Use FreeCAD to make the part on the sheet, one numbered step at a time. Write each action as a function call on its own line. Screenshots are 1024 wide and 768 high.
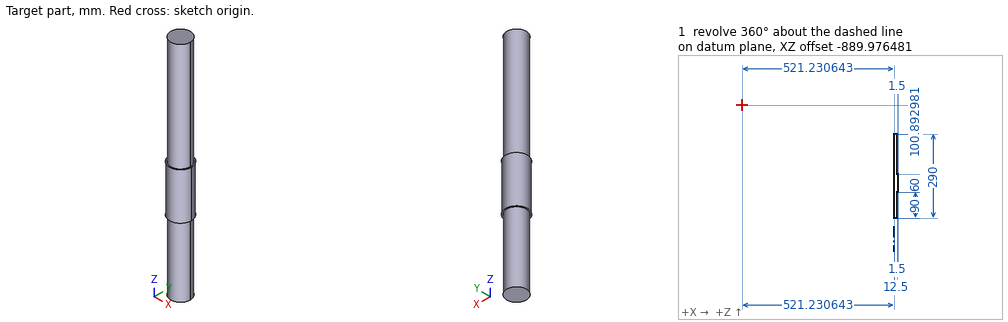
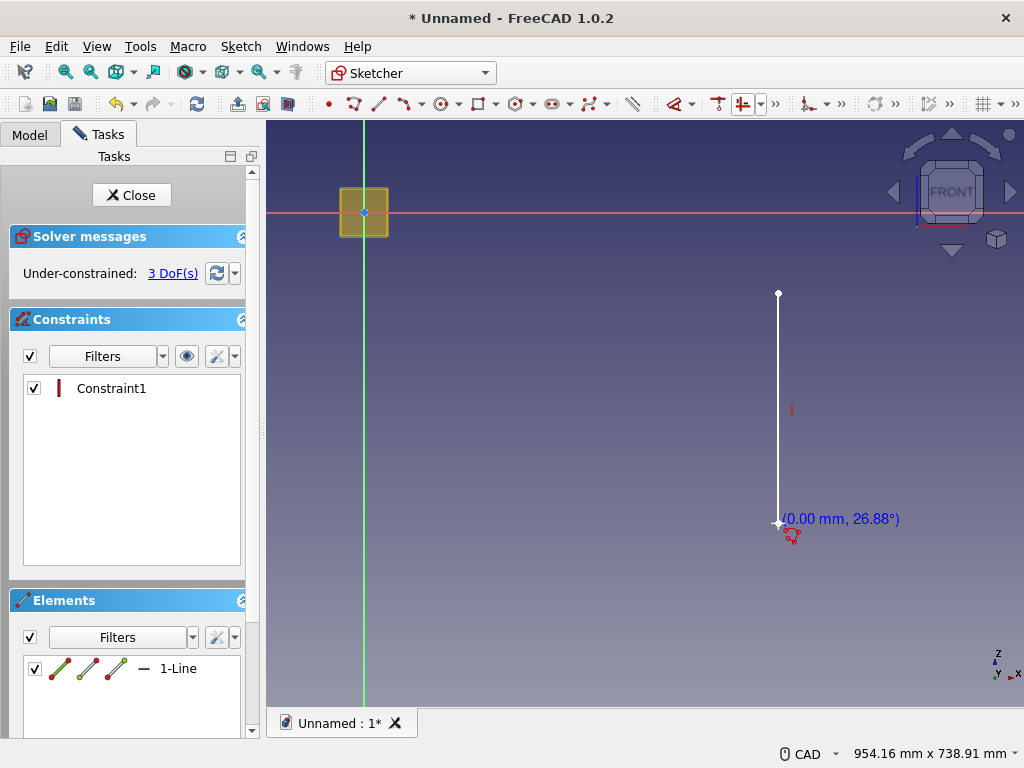
scroll(788, 523, up, 3)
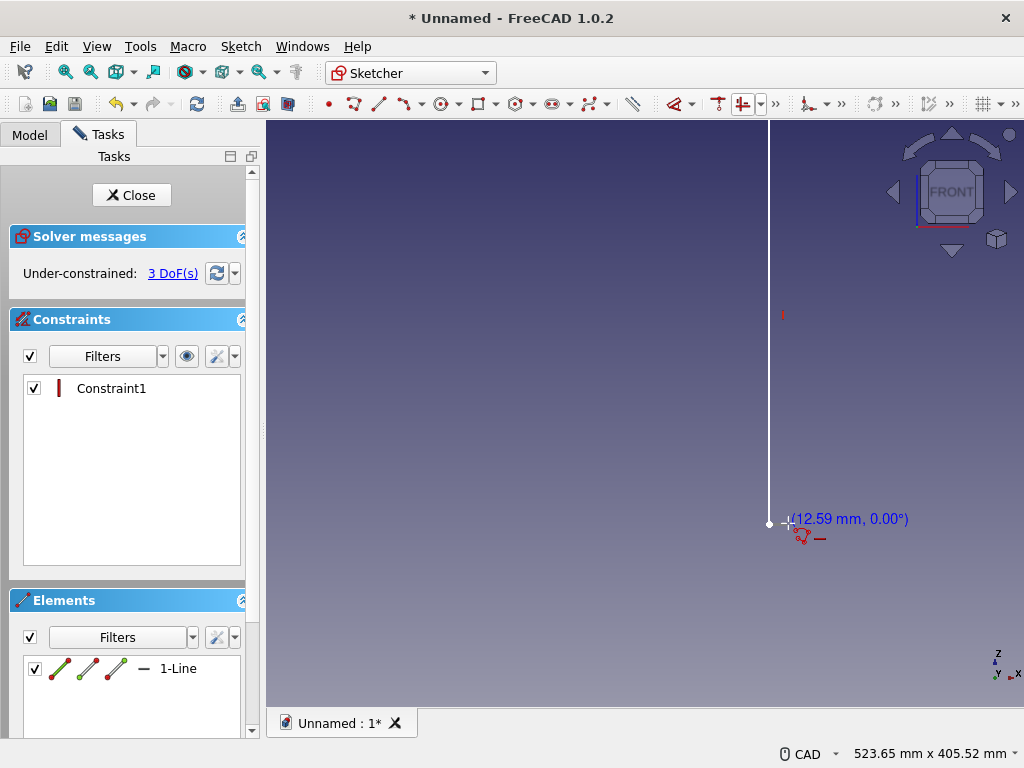
click(788, 522)
click(788, 392)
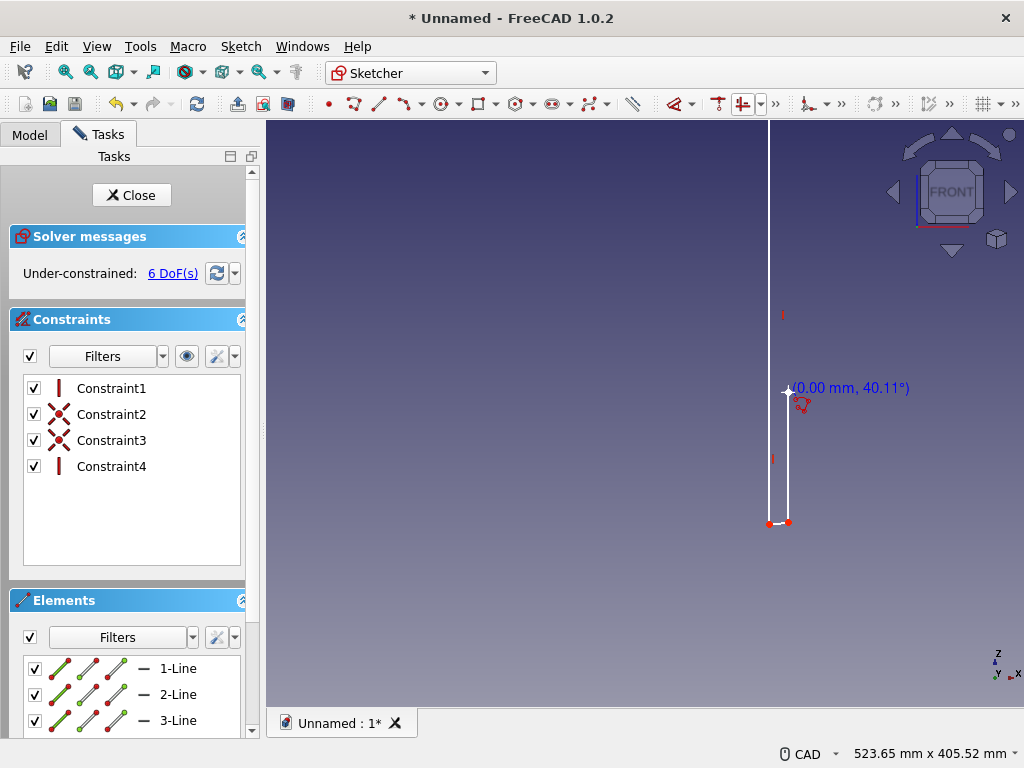
scroll(790, 392, up, 10)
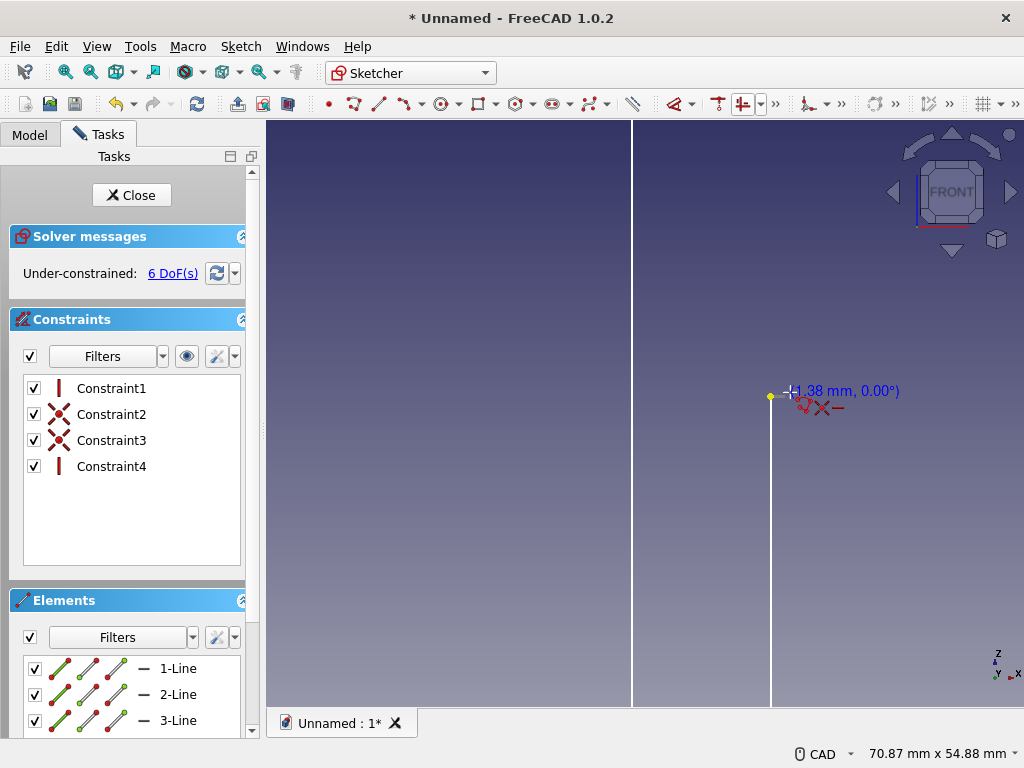
click(783, 389)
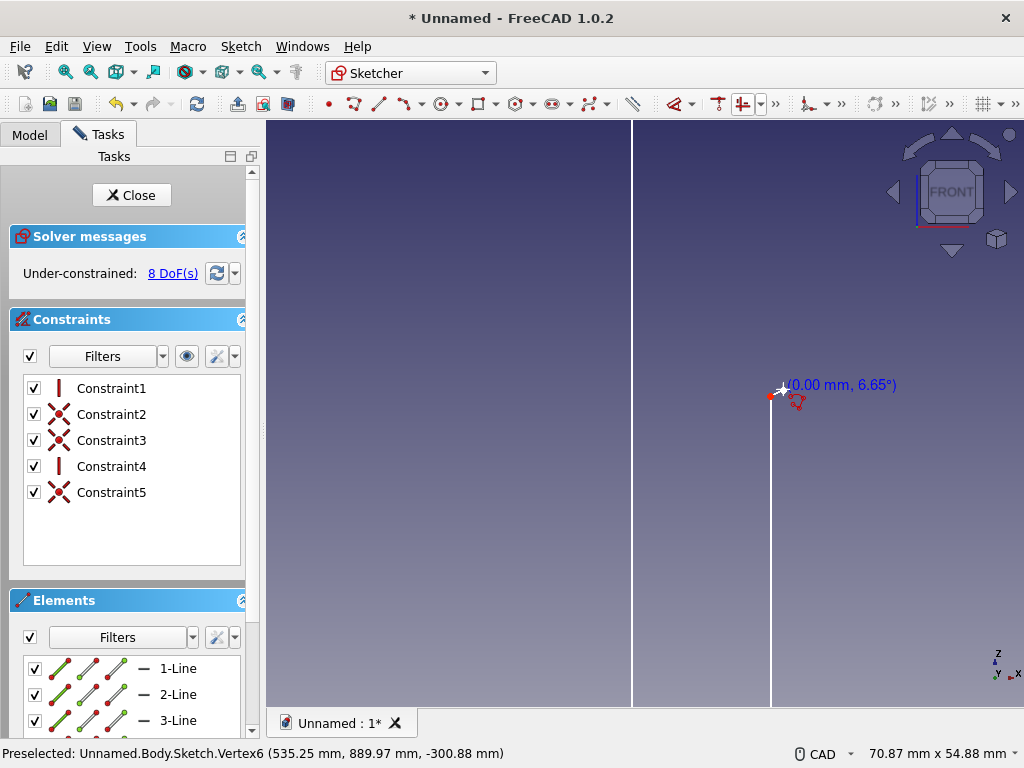
scroll(790, 456, down, 13)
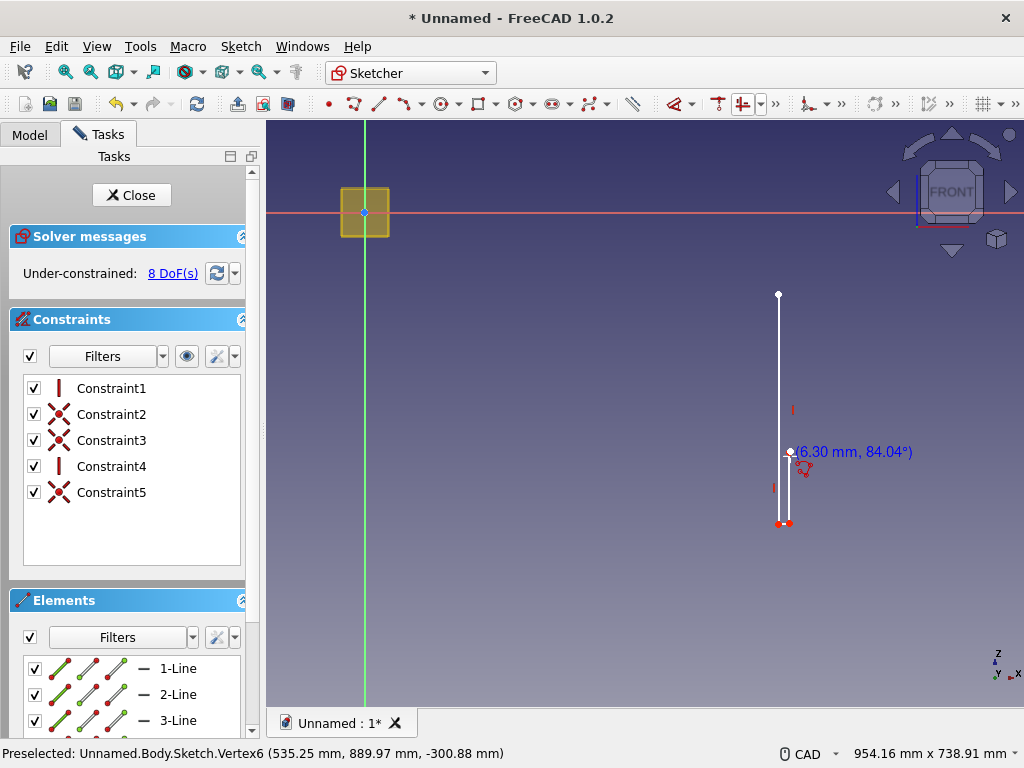
scroll(790, 404, up, 2)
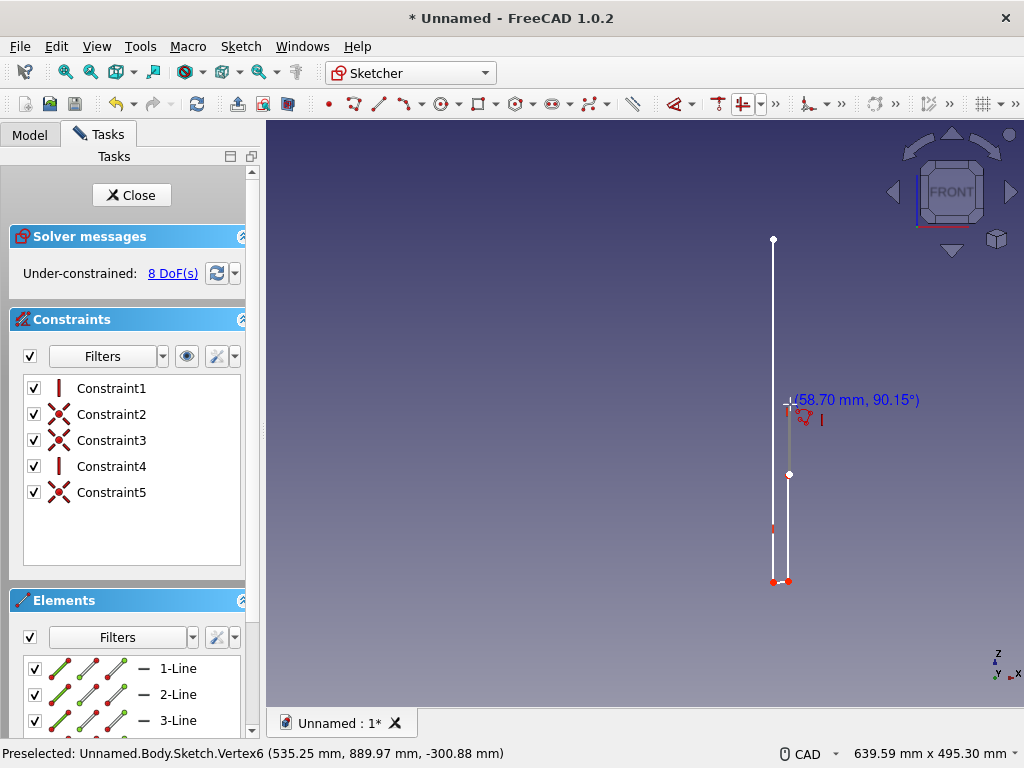
click(790, 404)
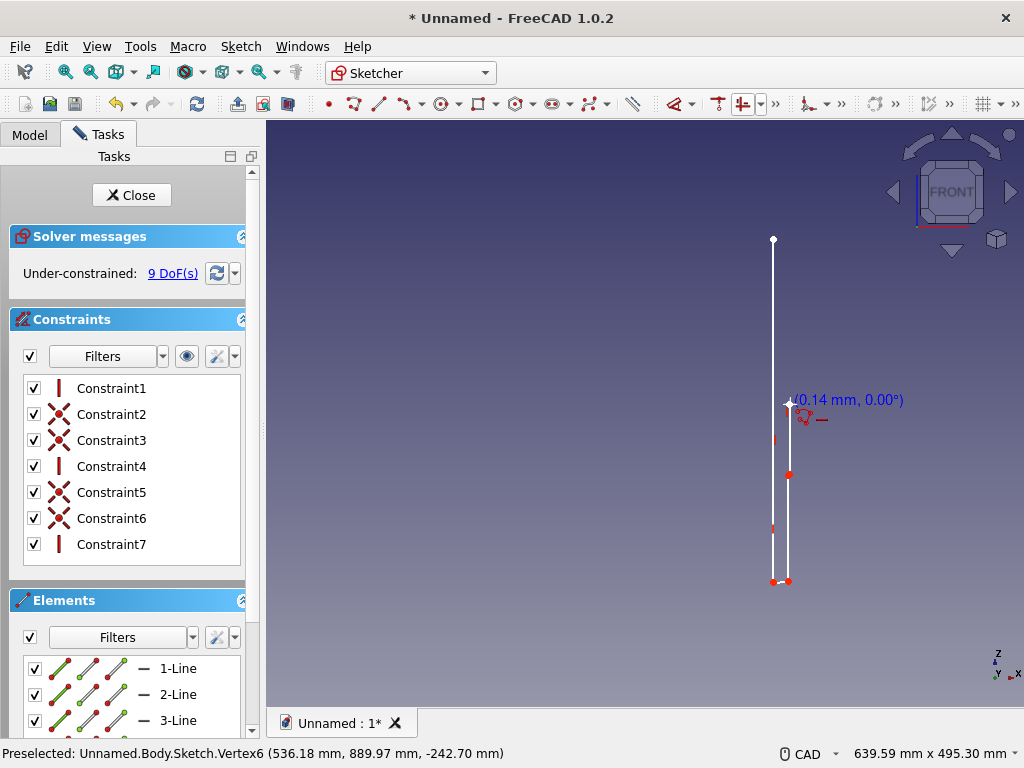
scroll(788, 404, up, 11)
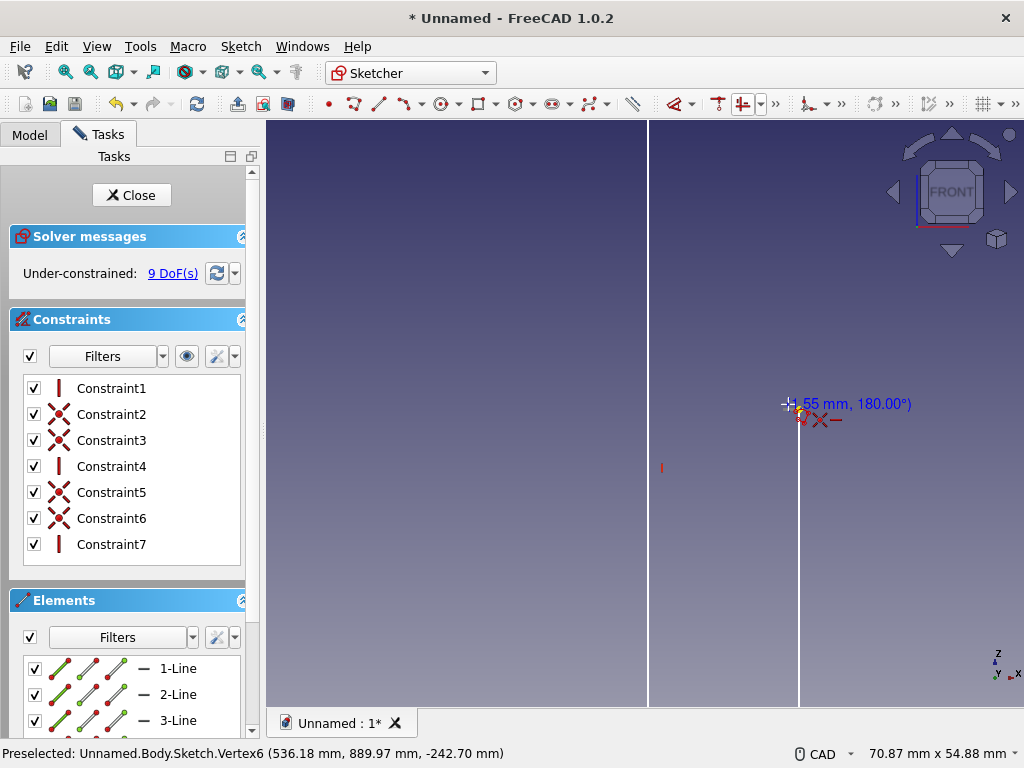
click(783, 400)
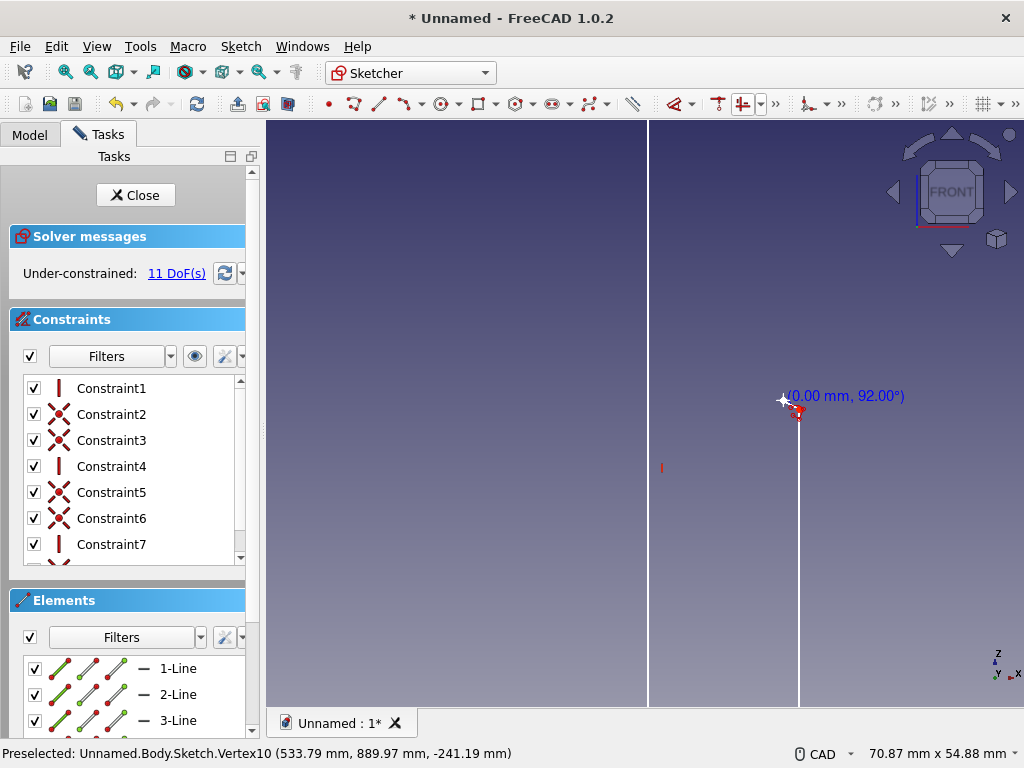
scroll(788, 404, down, 13)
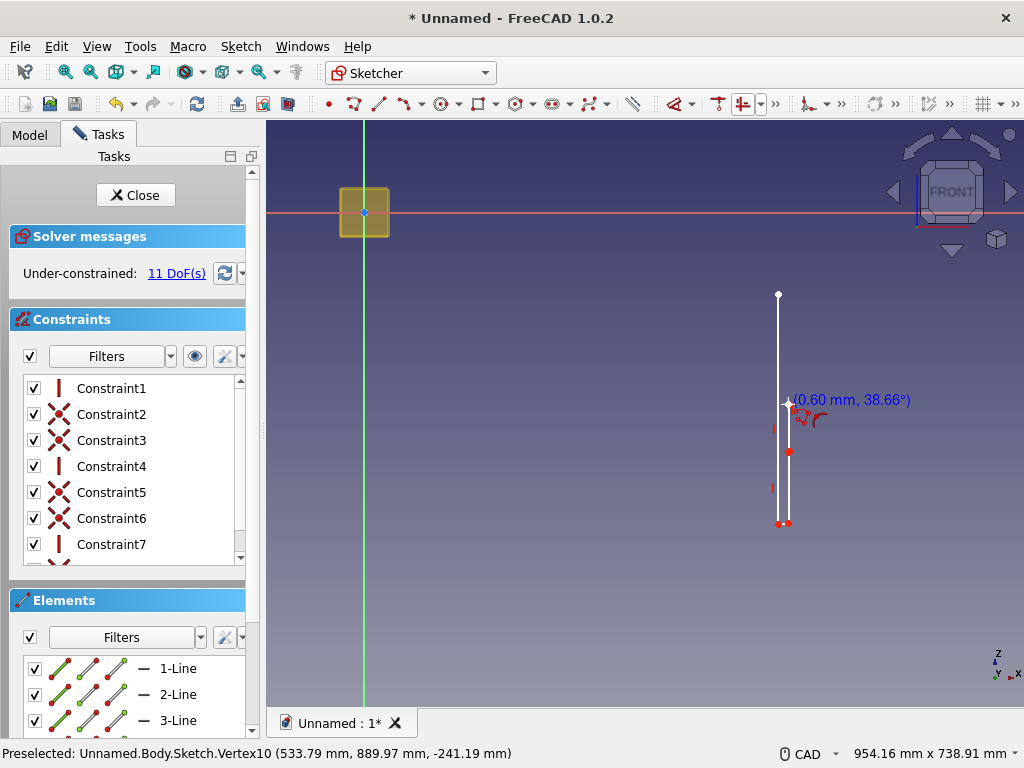
scroll(788, 293, up, 3)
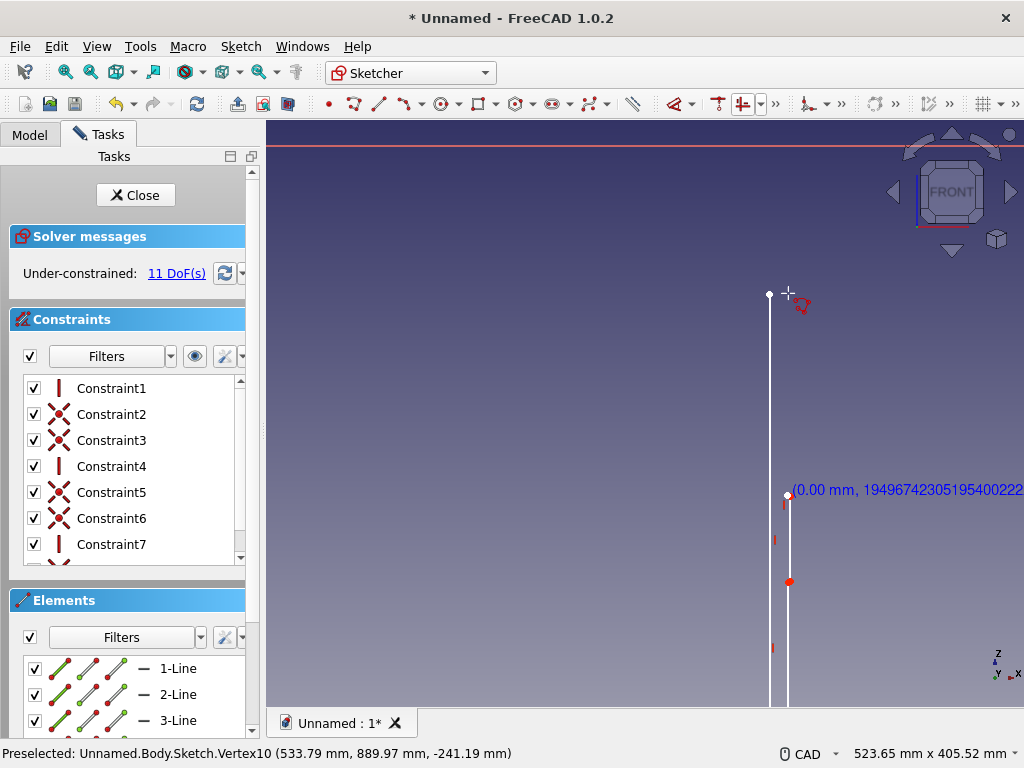
click(788, 292)
click(770, 295)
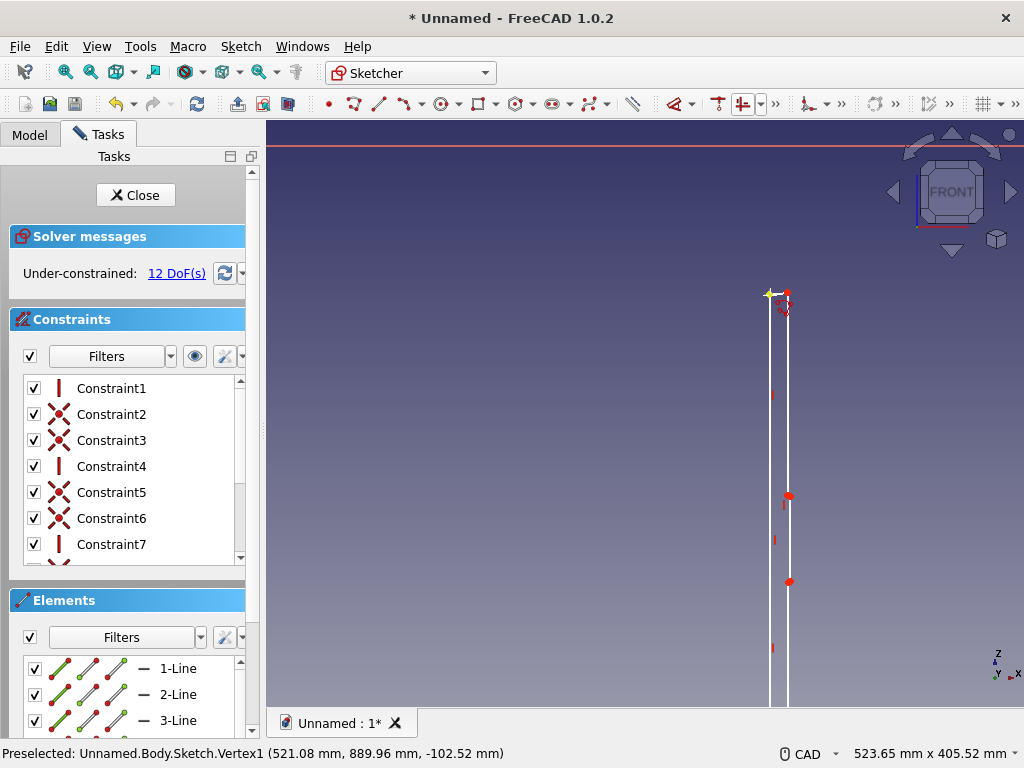
click(379, 104)